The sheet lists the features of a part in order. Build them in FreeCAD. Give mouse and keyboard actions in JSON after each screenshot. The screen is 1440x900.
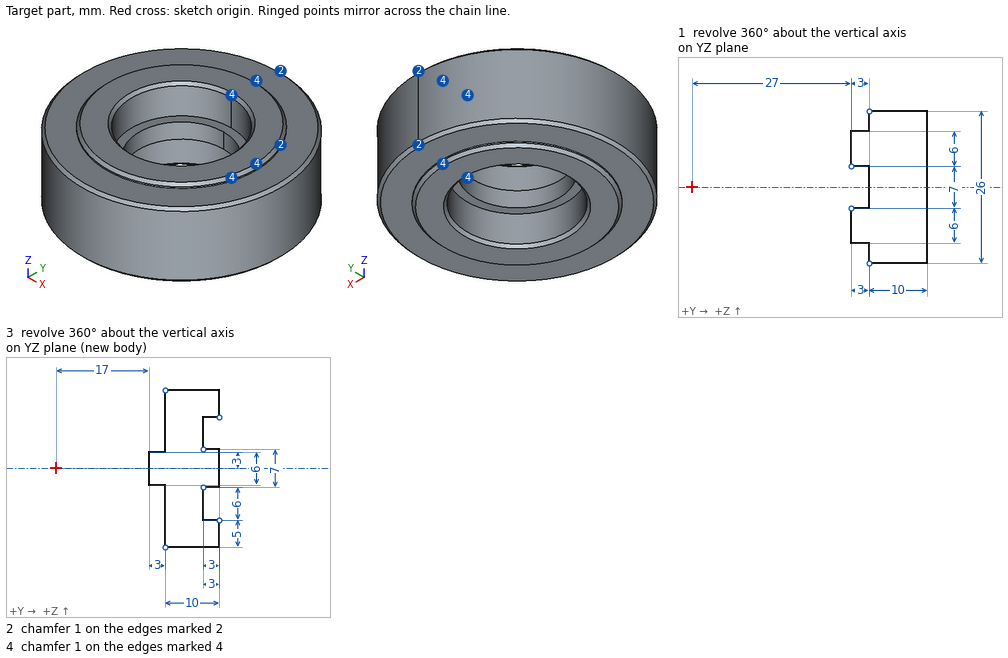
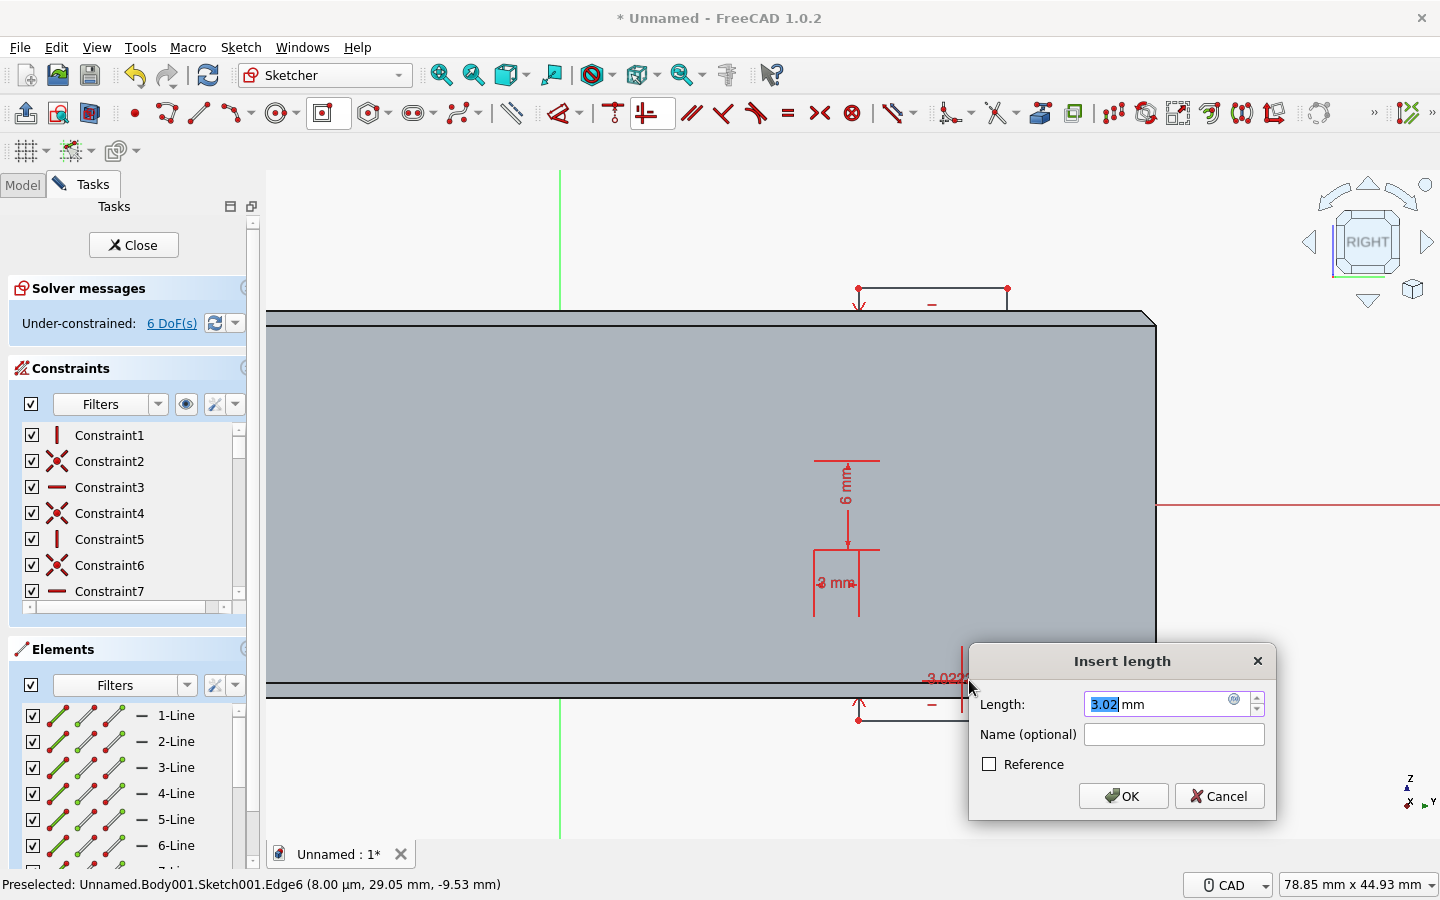
{"action": "type", "text": "3"}
{"action": "key", "text": "Return"}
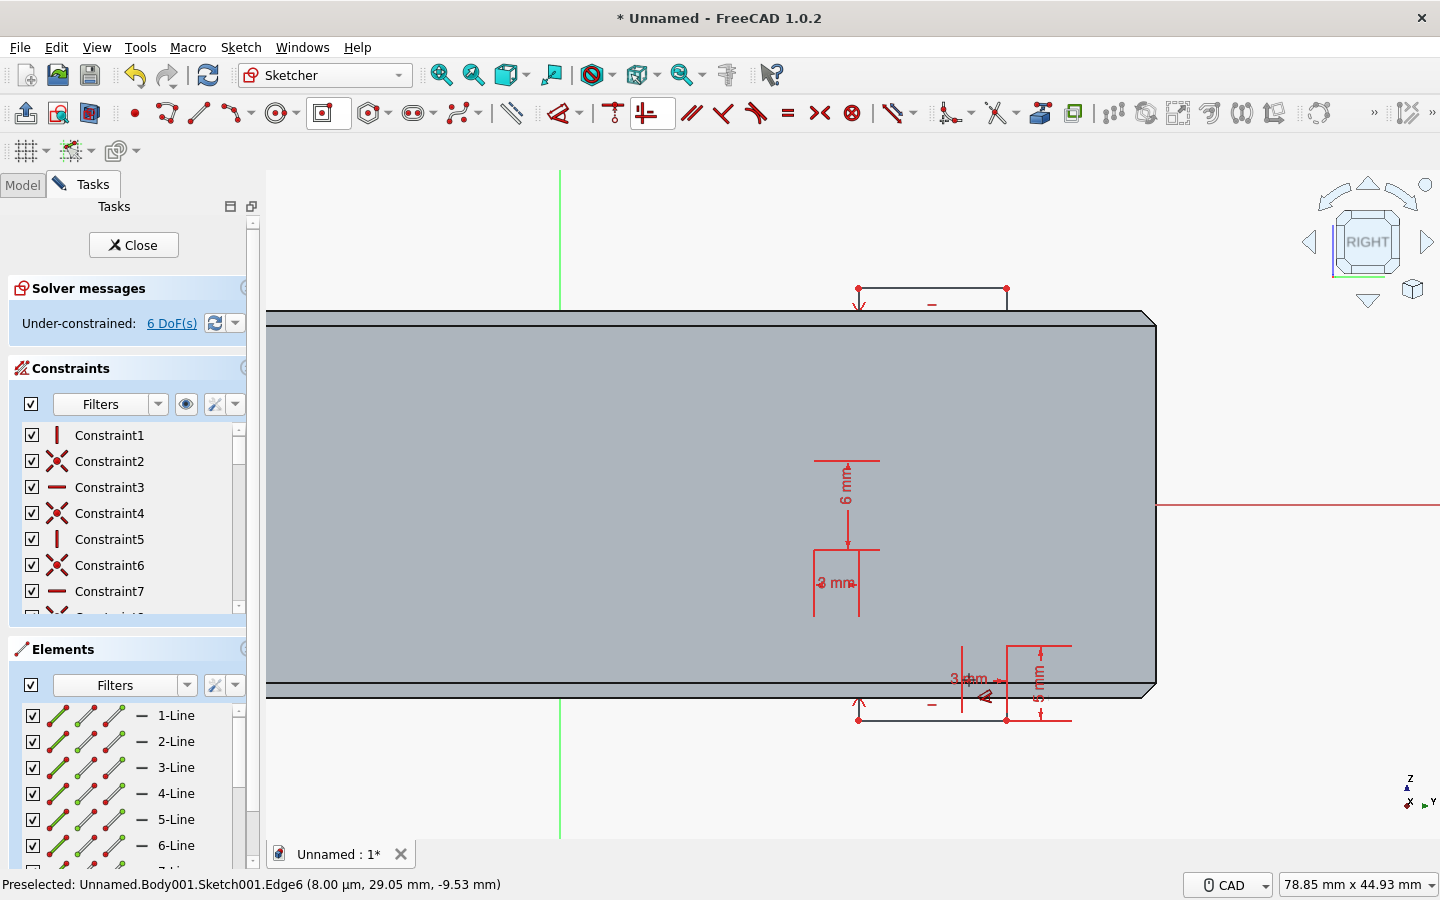
{"action": "left_click", "coordinate": [962, 619]}
{"action": "left_click", "coordinate": [996, 601]}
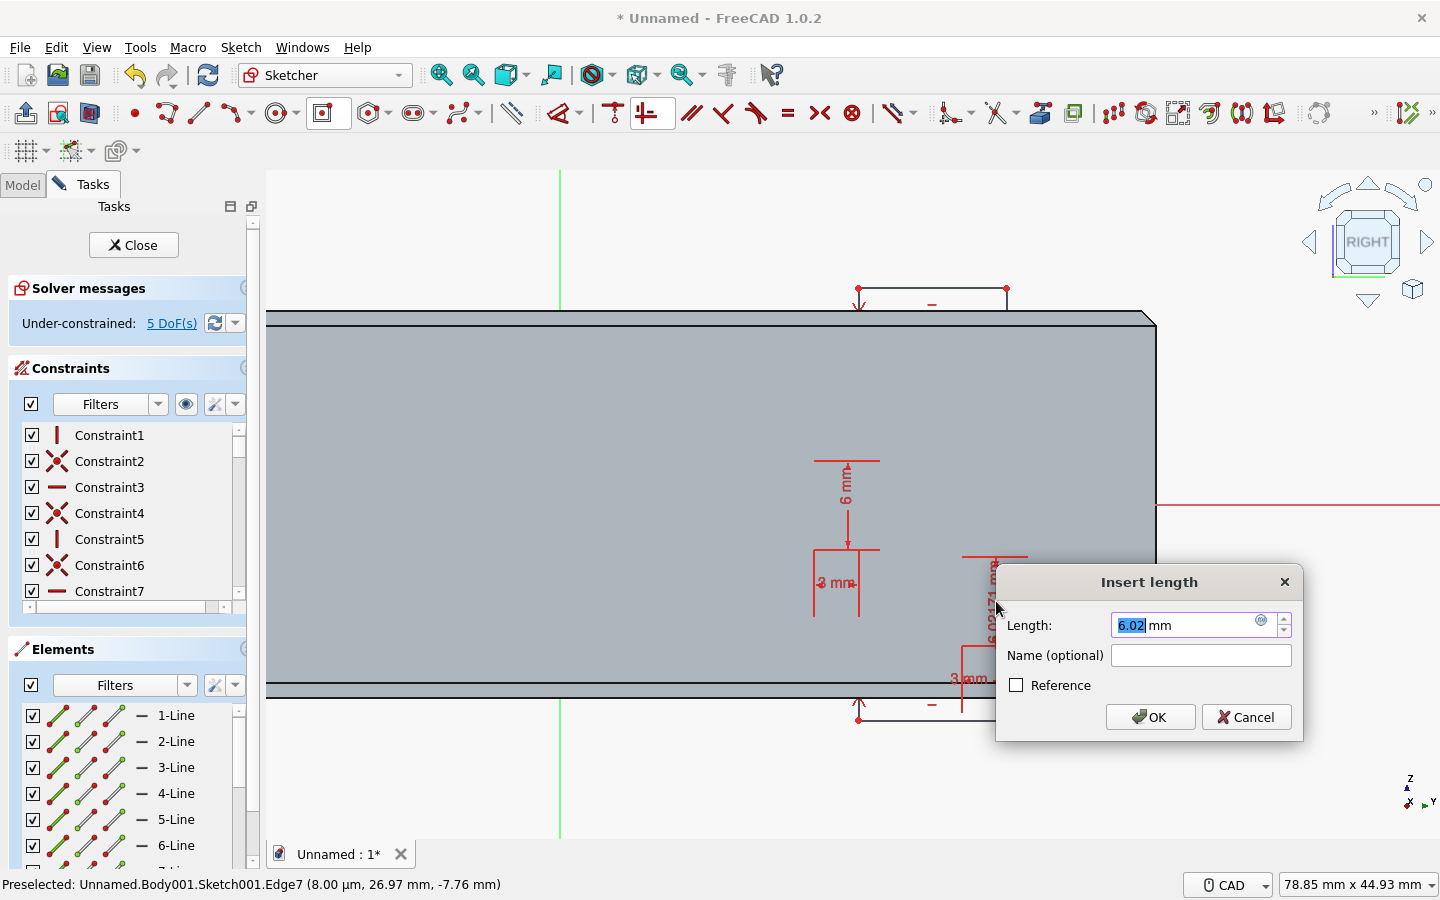
{"action": "type", "text": "6"}
{"action": "key", "text": "Return"}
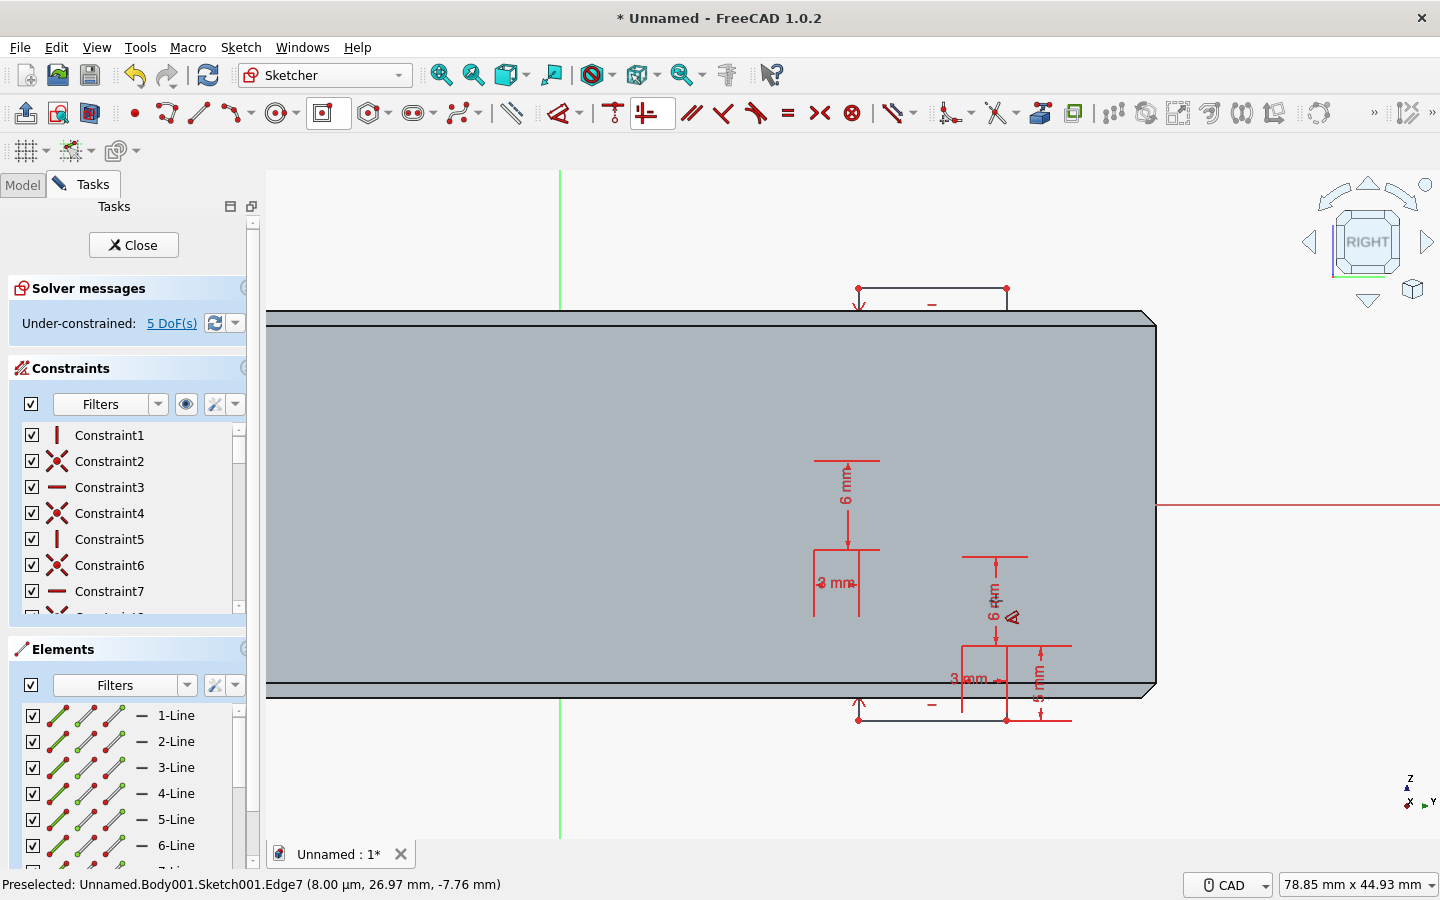
{"action": "left_click", "coordinate": [975, 557]}
{"action": "left_click", "coordinate": [984, 523]}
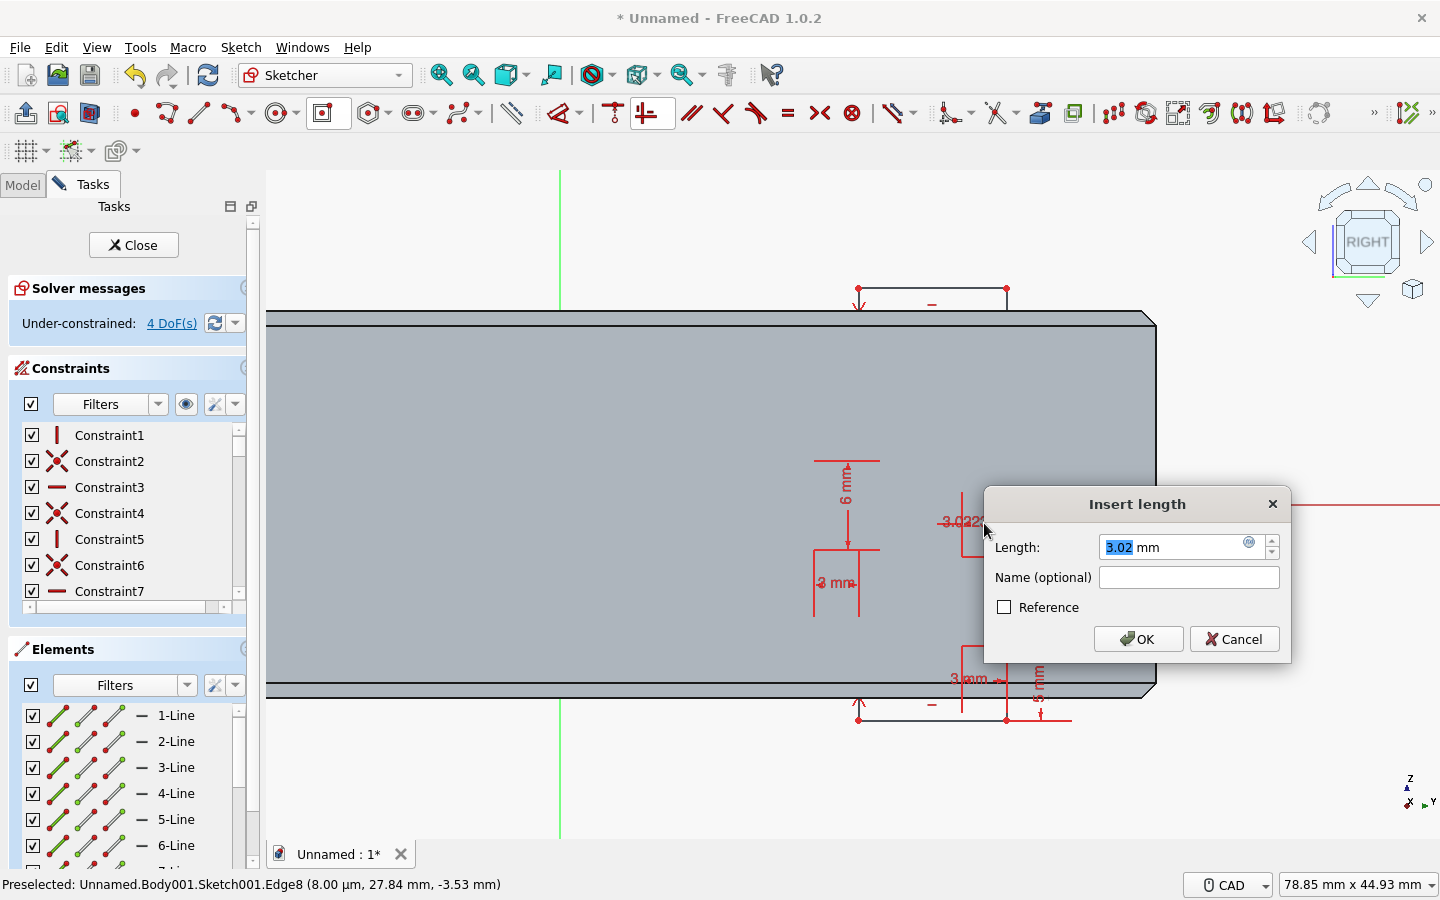
{"action": "type", "text": "3"}
{"action": "key", "text": "Return"}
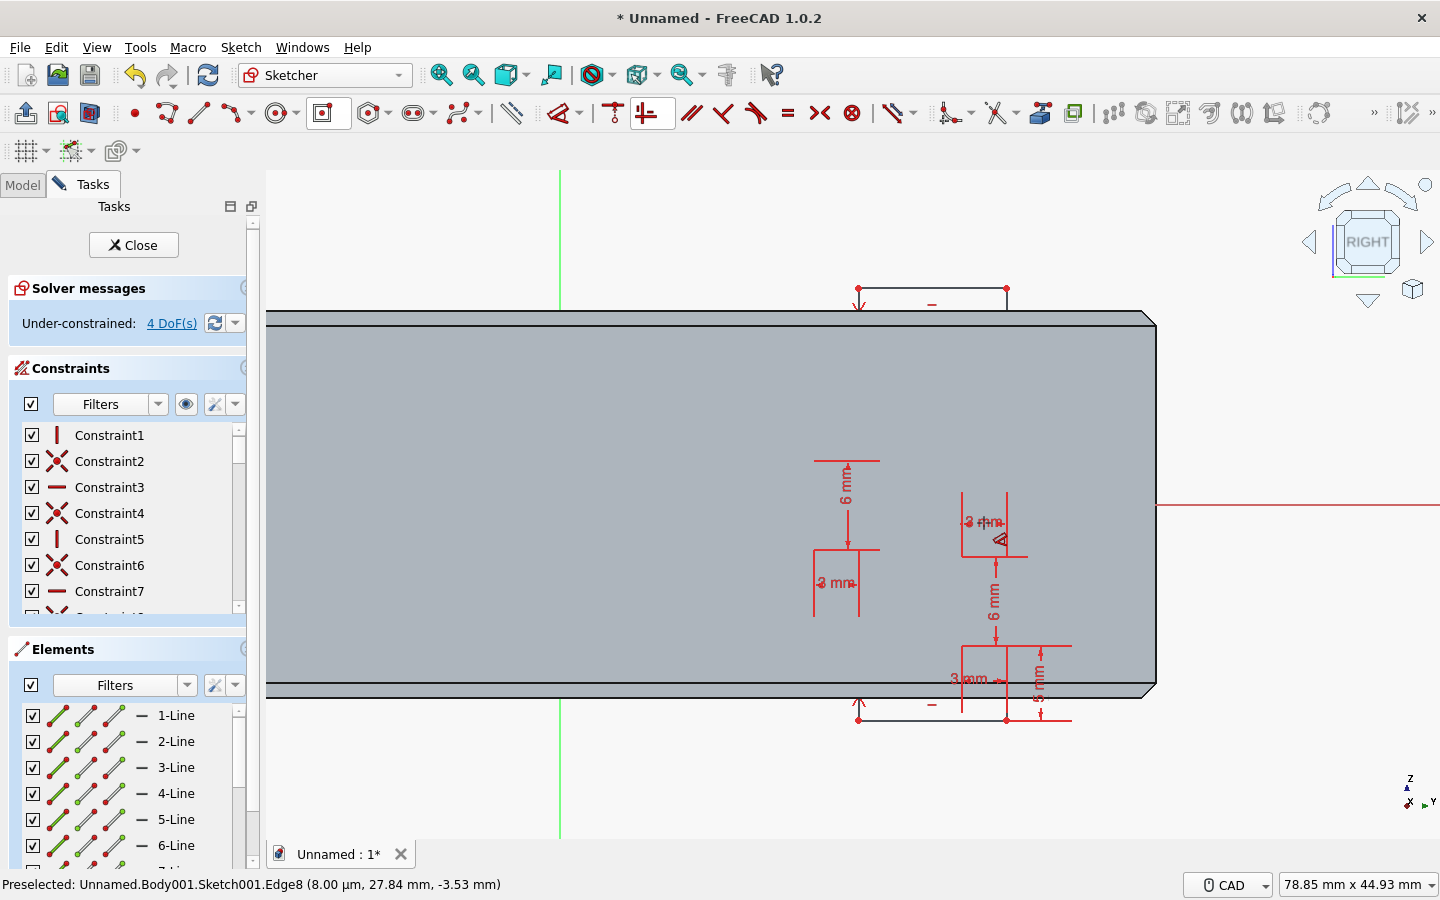
{"action": "left_click", "coordinate": [1007, 525]}
{"action": "left_click", "coordinate": [1041, 480]}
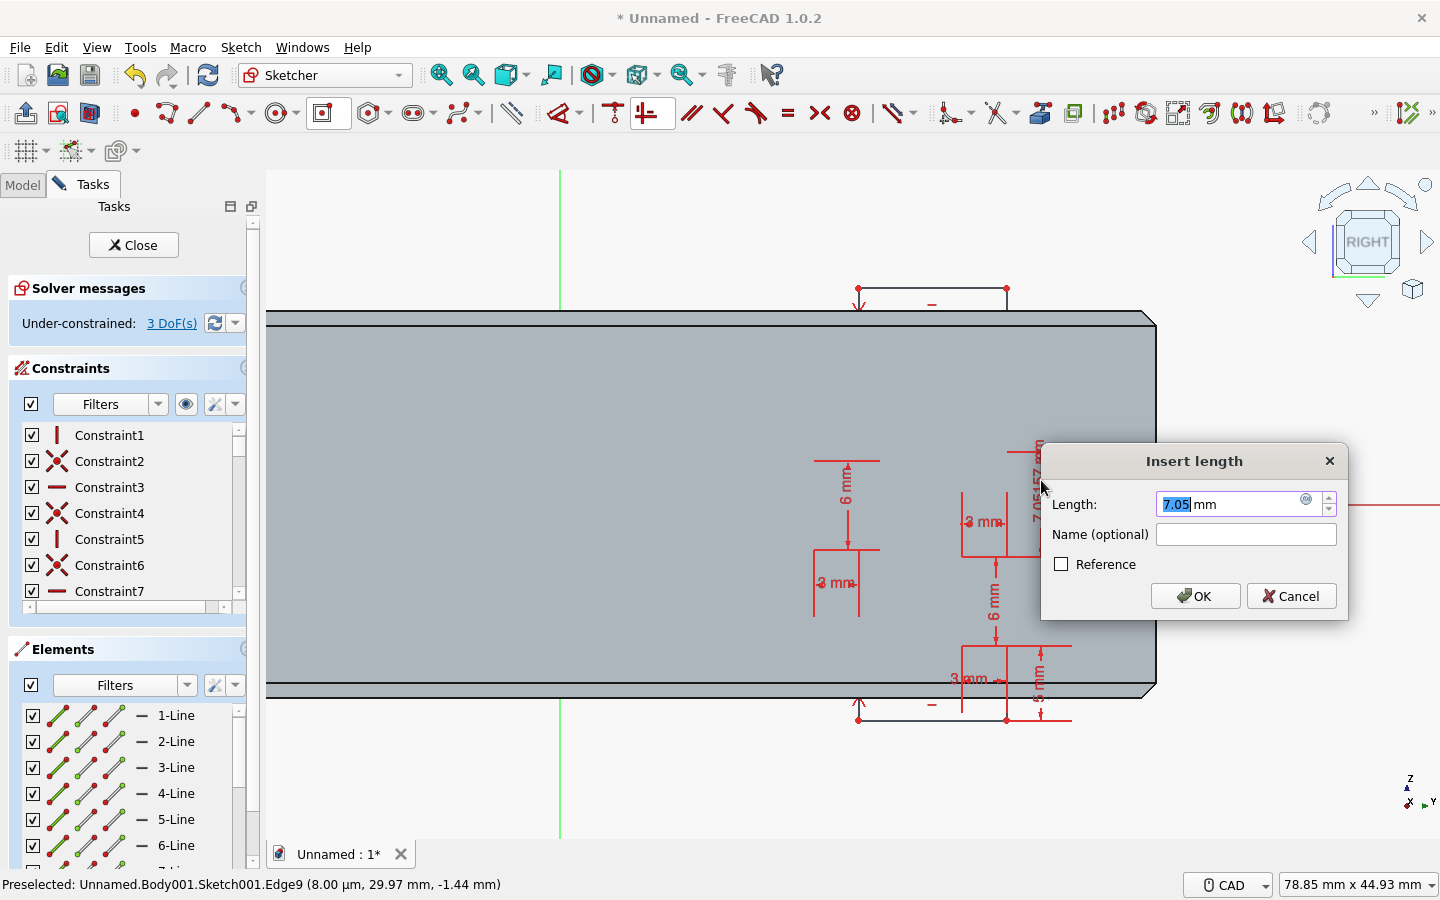
{"action": "type", "text": "7"}
{"action": "key", "text": "Return"}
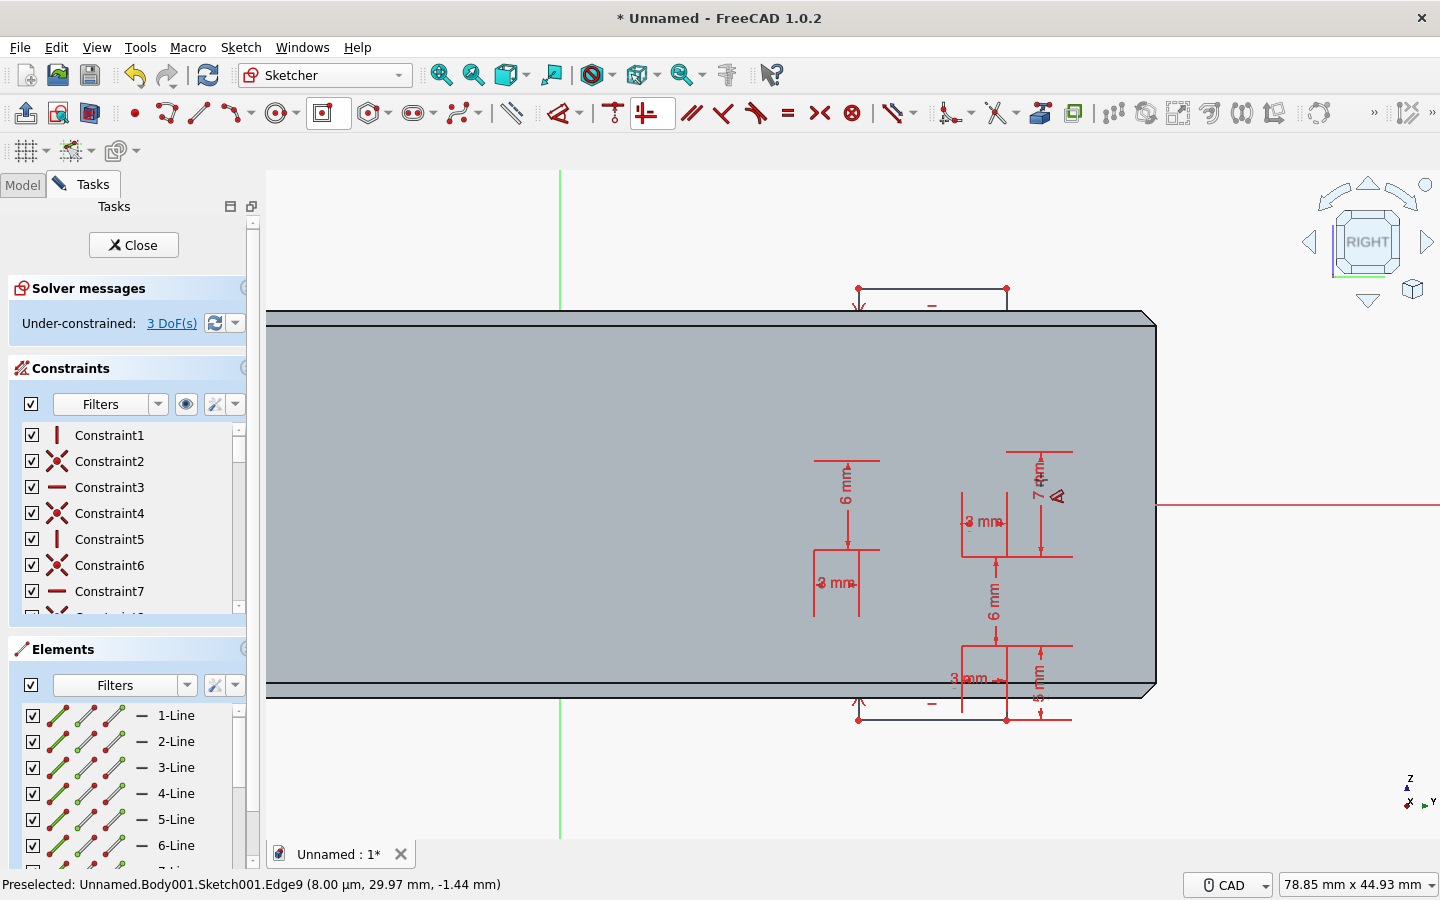
{"action": "left_click", "coordinate": [903, 720]}
{"action": "left_click", "coordinate": [933, 754]}